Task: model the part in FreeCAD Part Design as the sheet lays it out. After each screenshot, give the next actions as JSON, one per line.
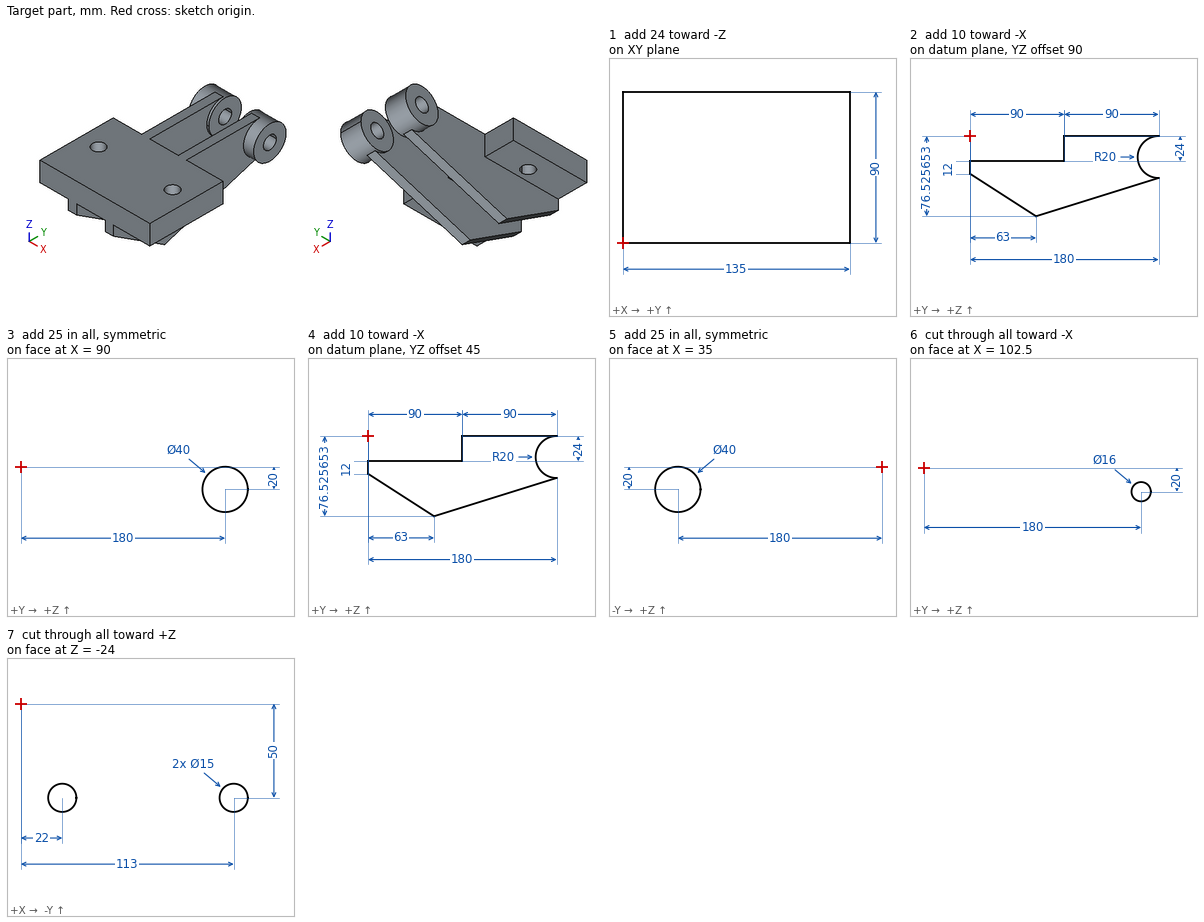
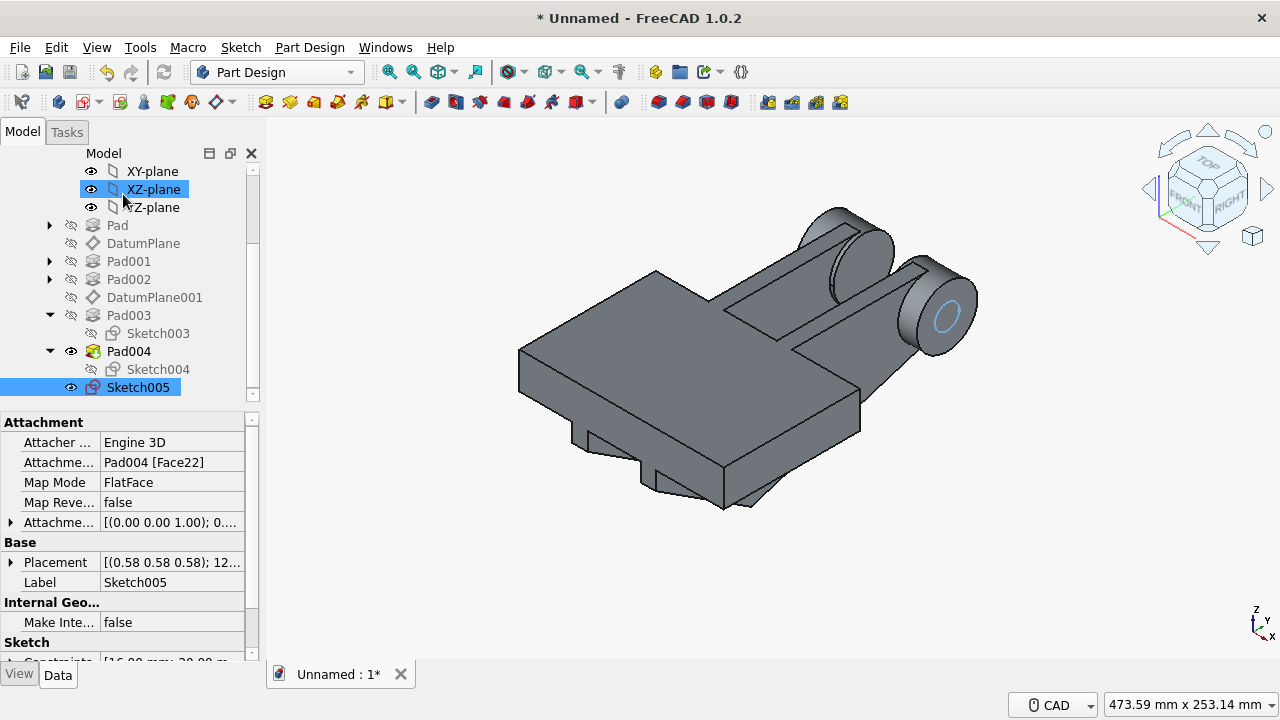
{"action": "left_click", "coordinate": [432, 102]}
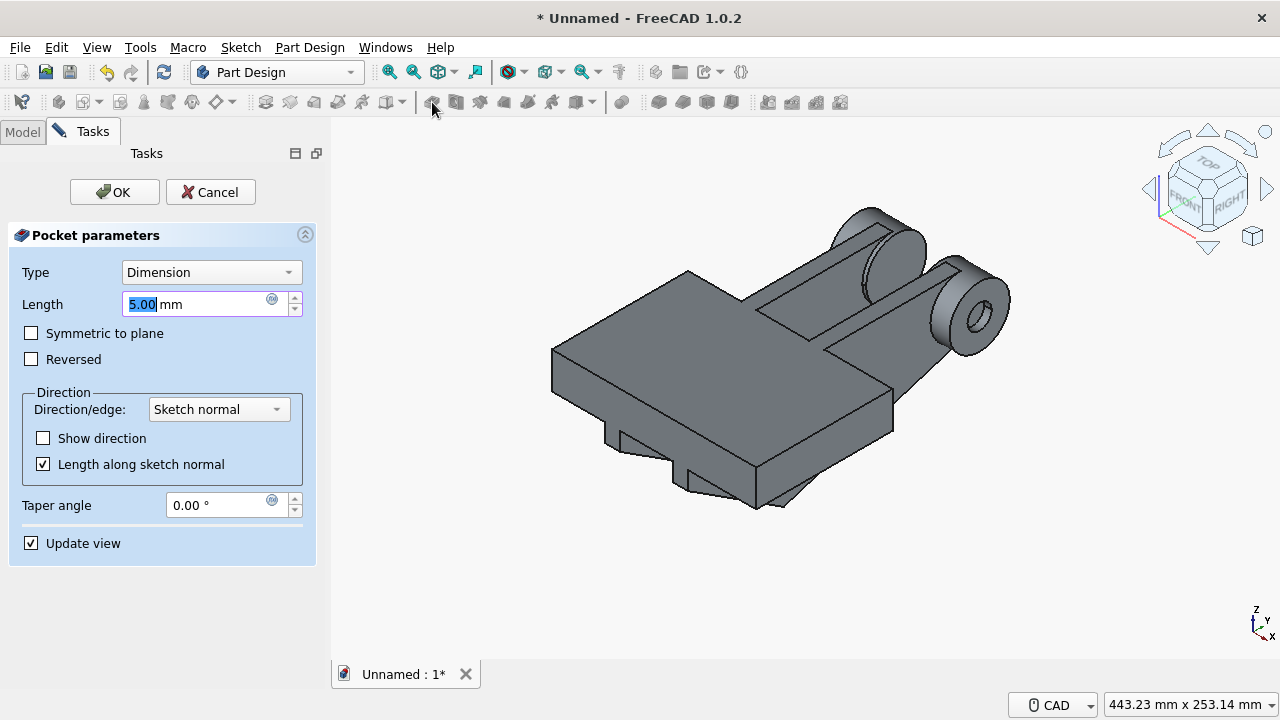
{"action": "left_click", "coordinate": [212, 272]}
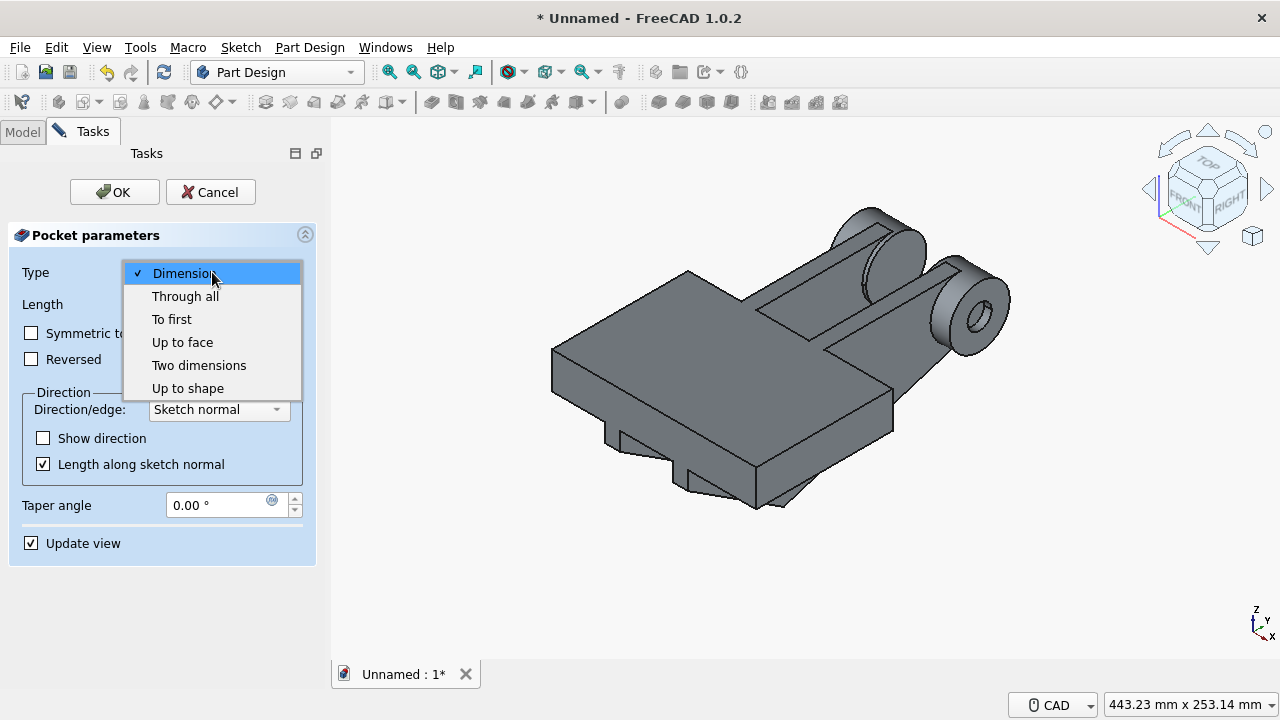
{"action": "left_click", "coordinate": [212, 296]}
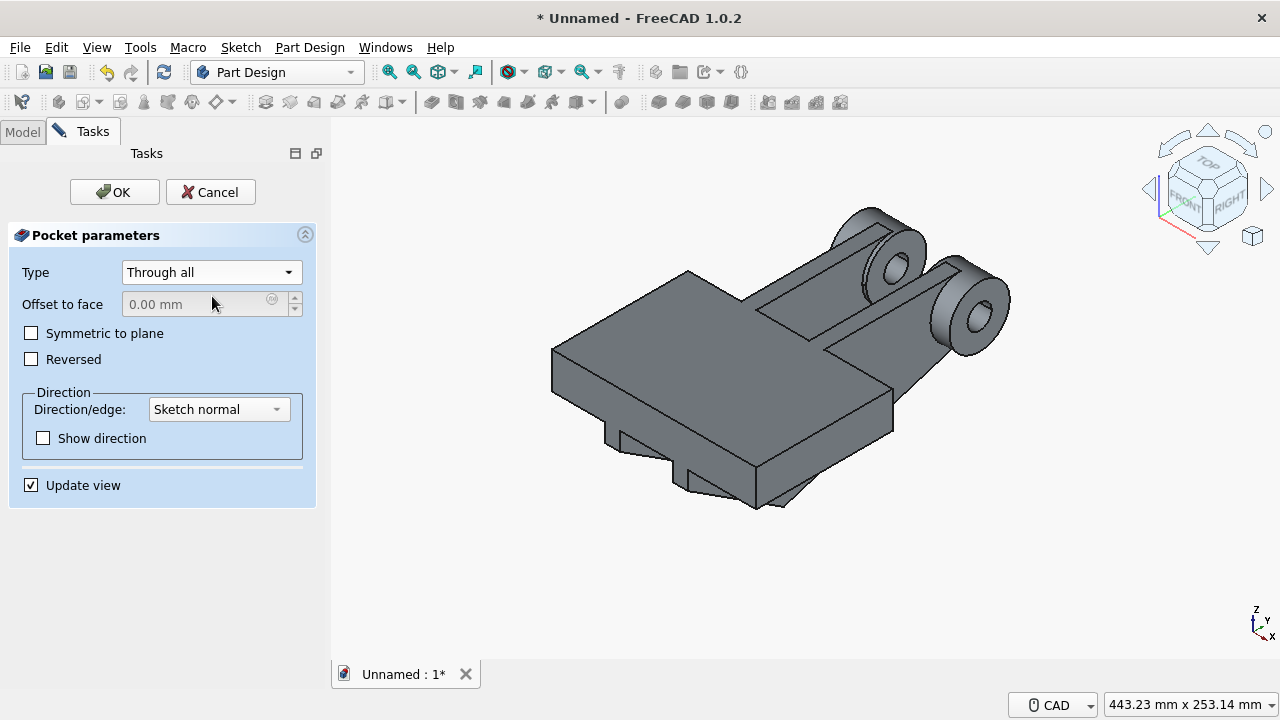
{"action": "left_click", "coordinate": [115, 192]}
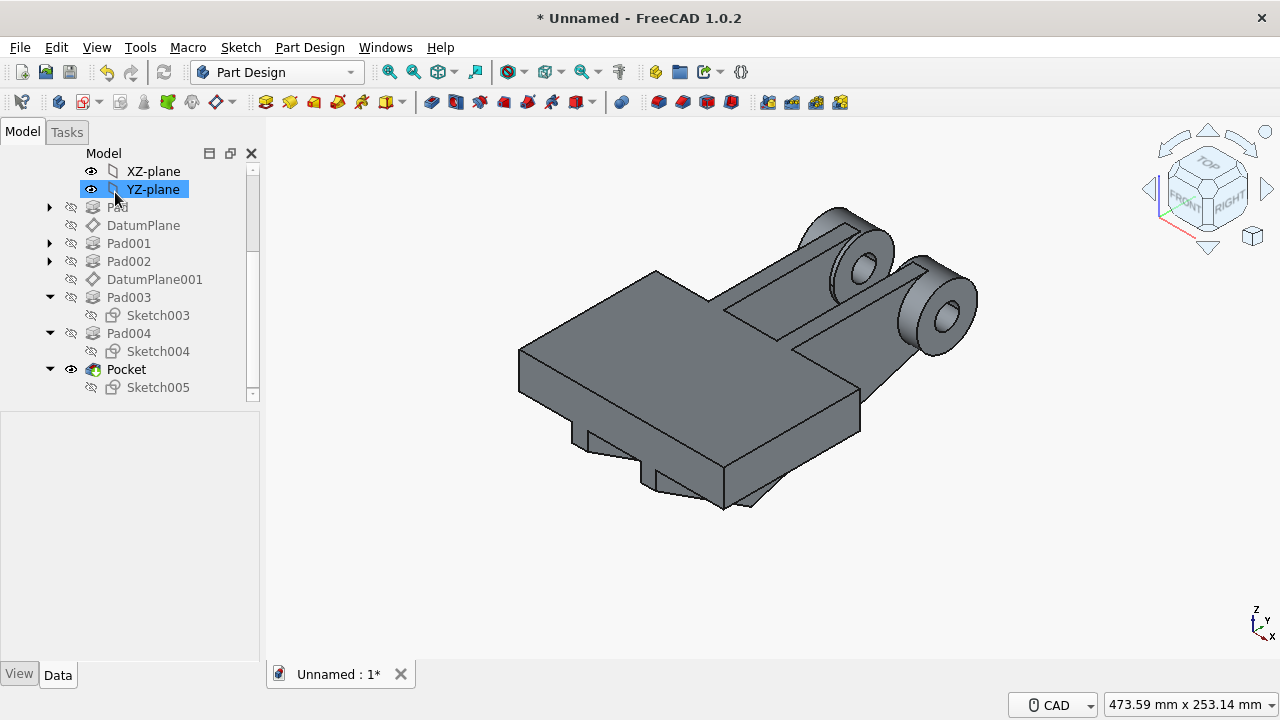
{"action": "key", "text": "5"}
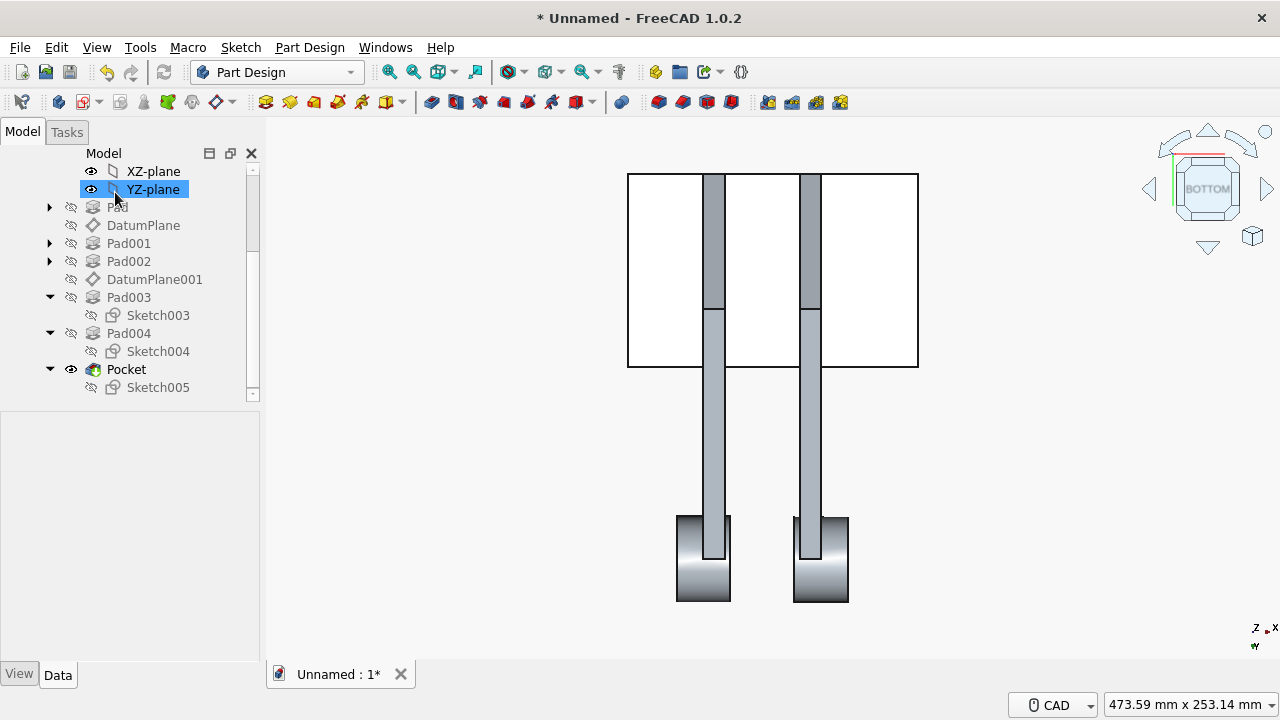
{"action": "left_click", "coordinate": [869, 297]}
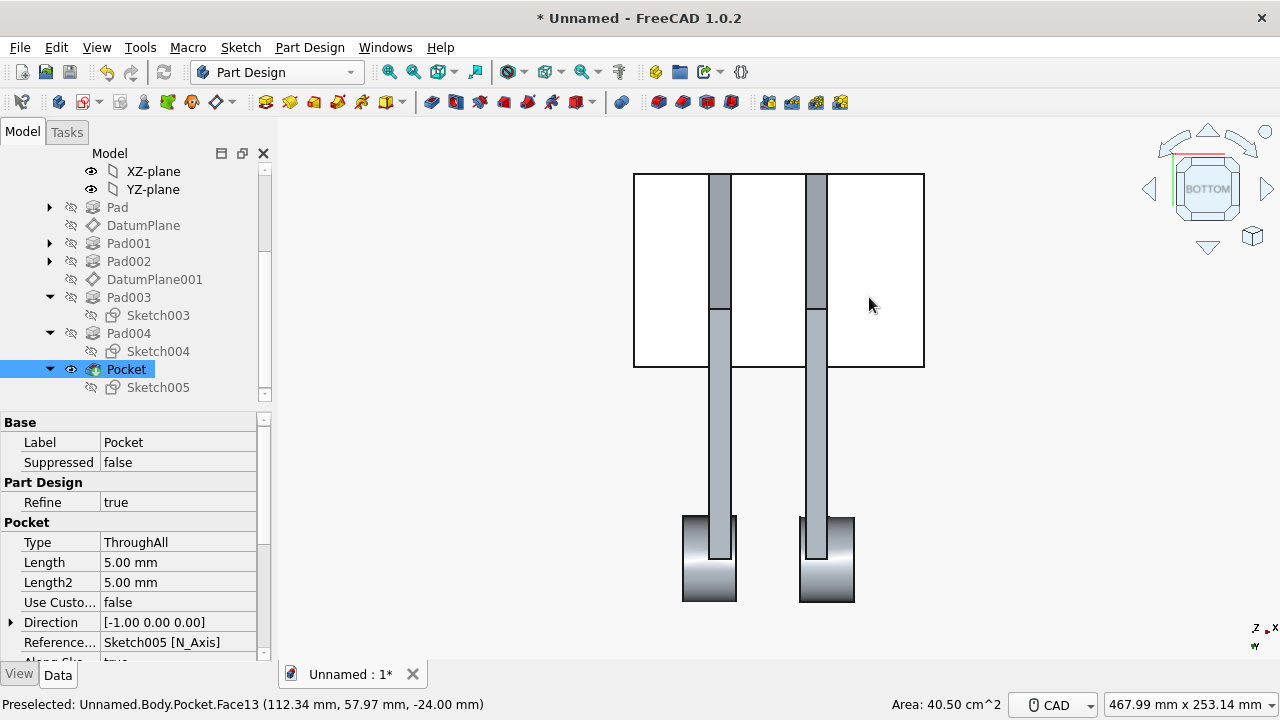
{"action": "left_click", "coordinate": [84, 102]}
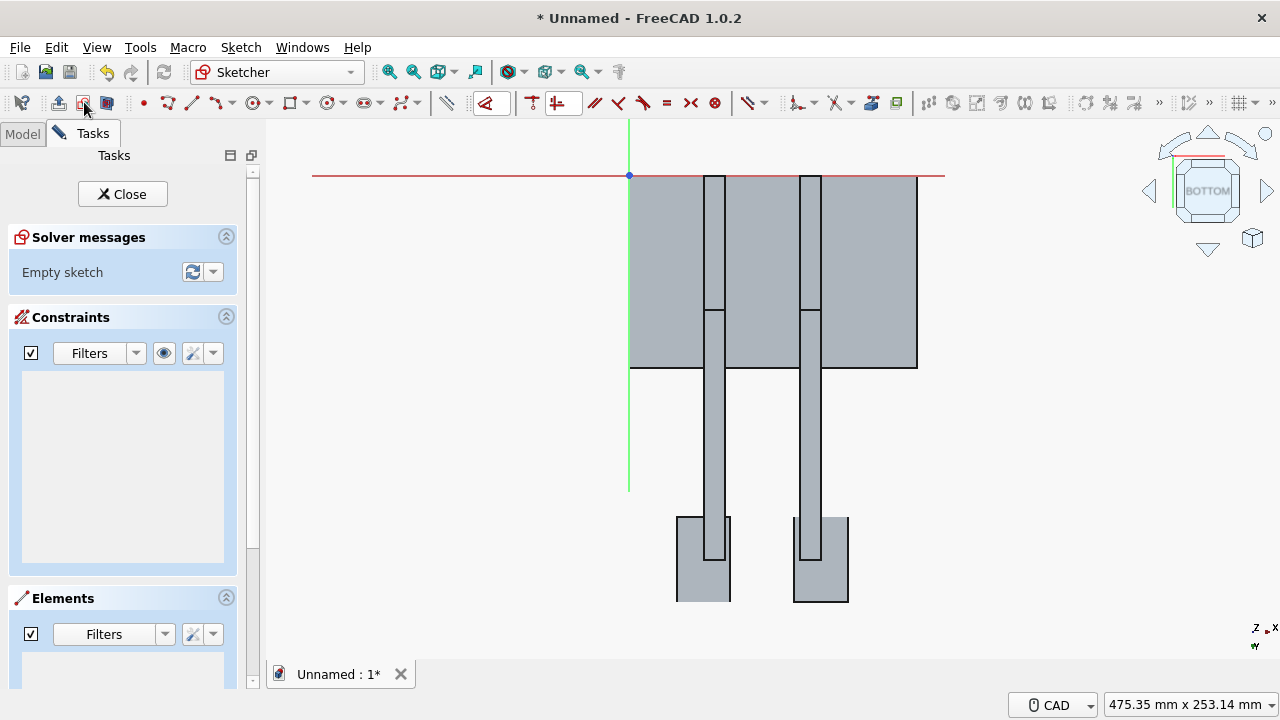
{"action": "left_click", "coordinate": [108, 104]}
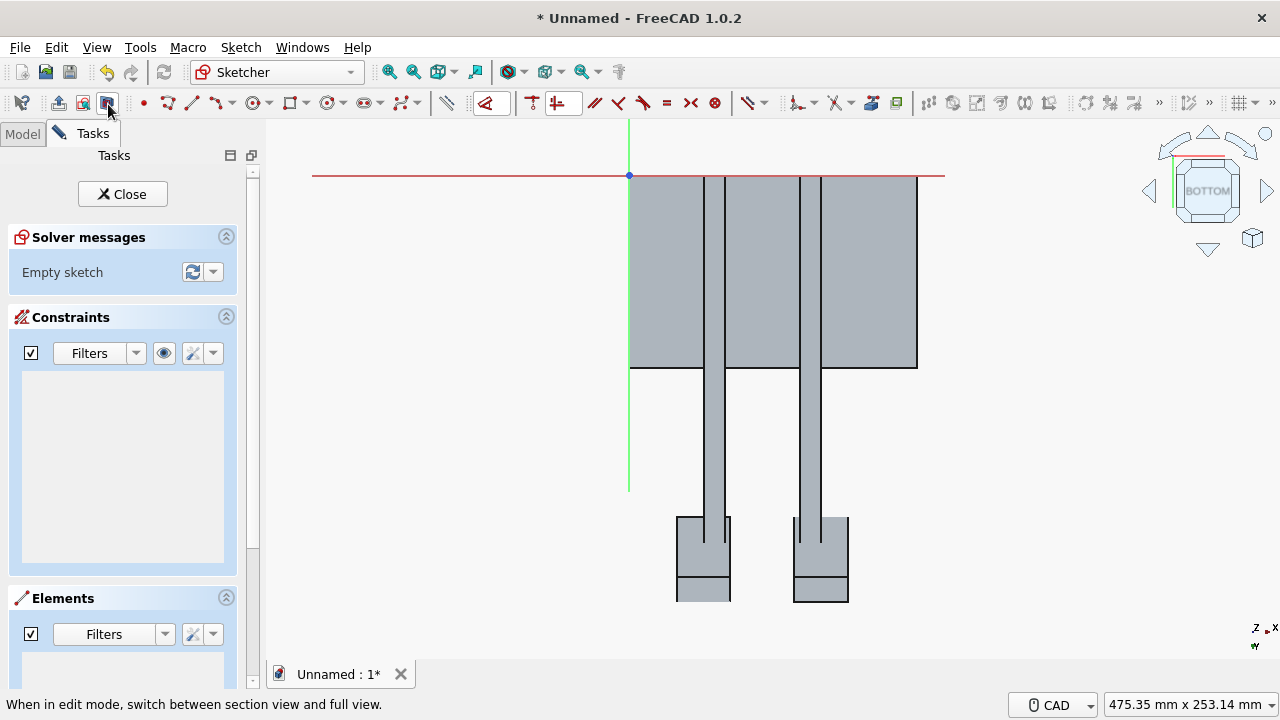
{"action": "scroll", "coordinate": [801, 147], "scroll_direction": "up", "scroll_amount": 4}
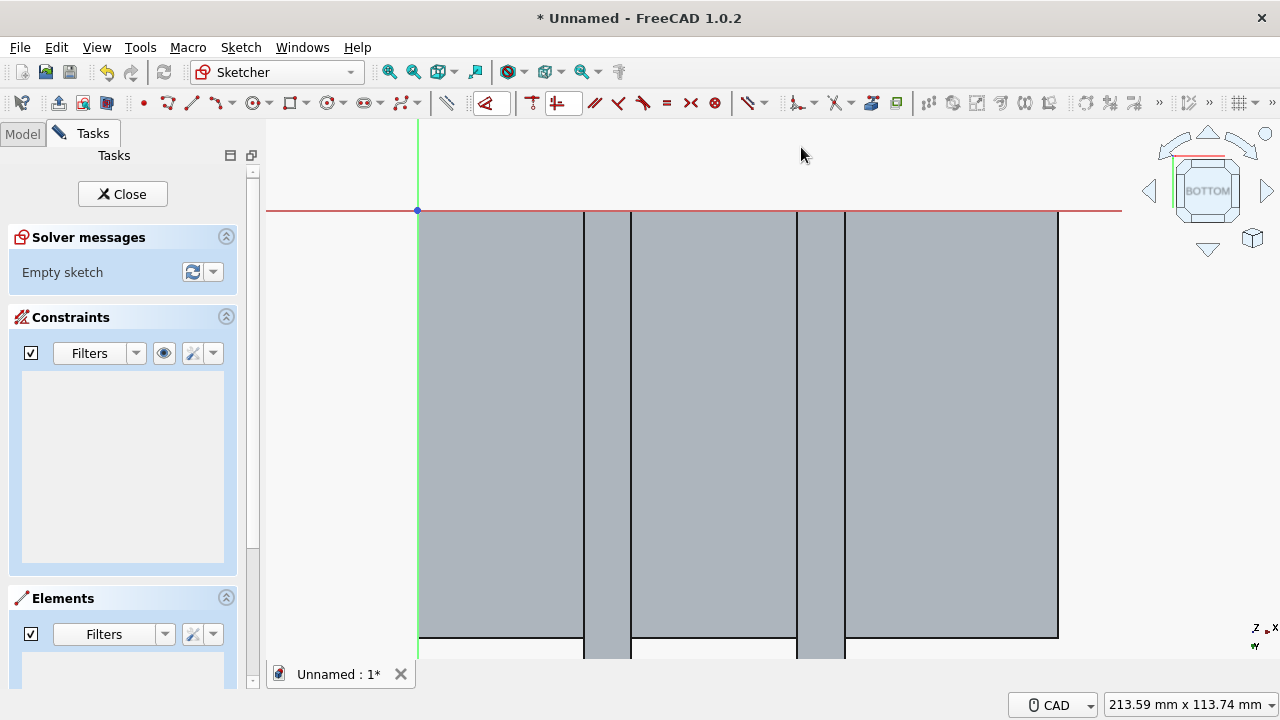
{"action": "left_click", "coordinate": [254, 104]}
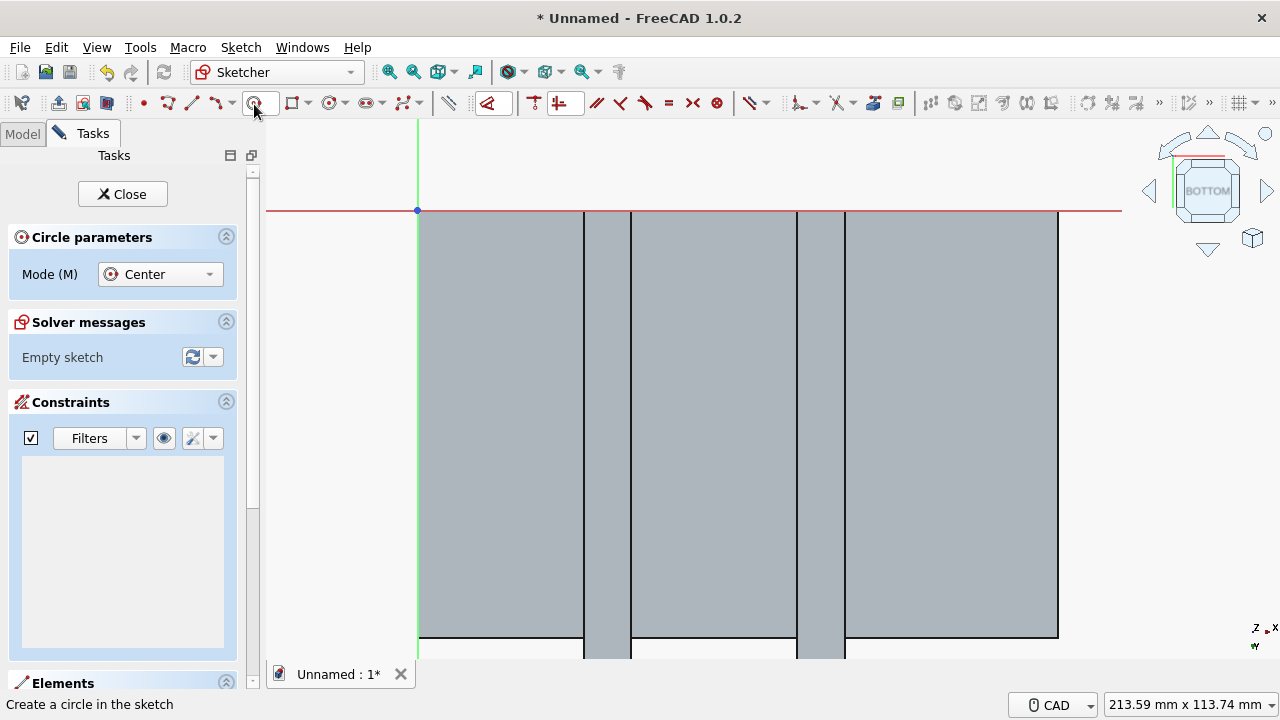
{"action": "left_click", "coordinate": [954, 448]}
{"action": "mouse_move", "coordinate": [979, 423]}